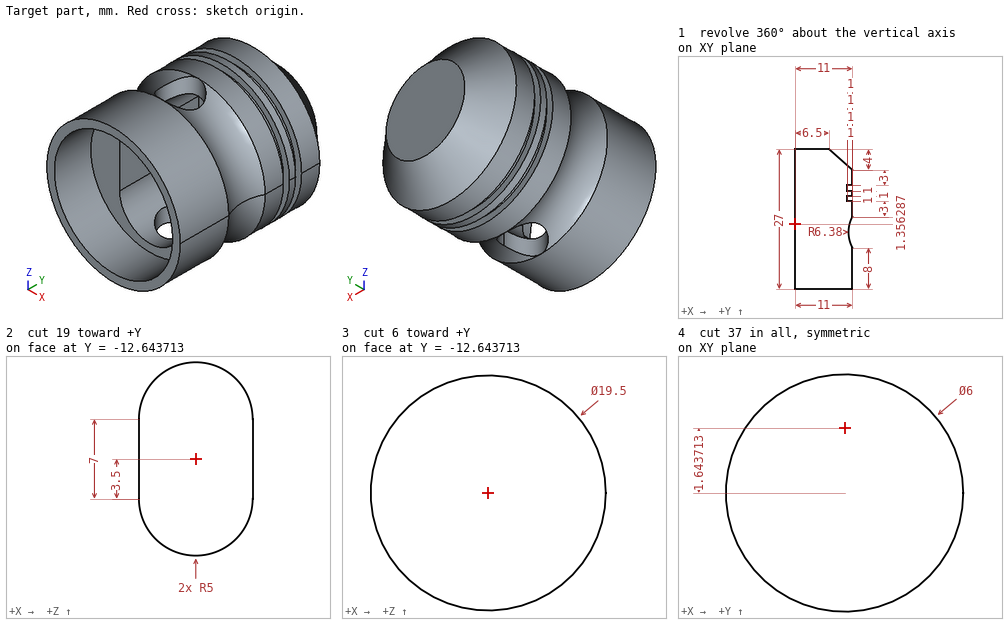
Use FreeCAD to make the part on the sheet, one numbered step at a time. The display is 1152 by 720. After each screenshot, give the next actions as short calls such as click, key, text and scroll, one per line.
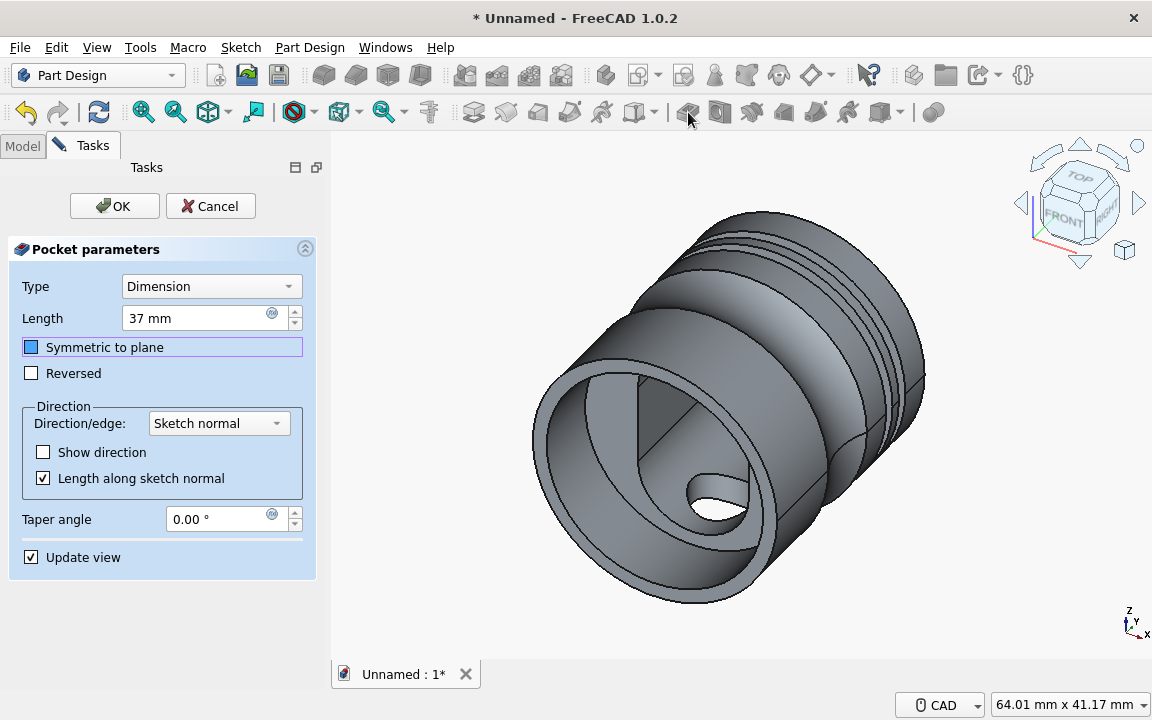
click(30, 347)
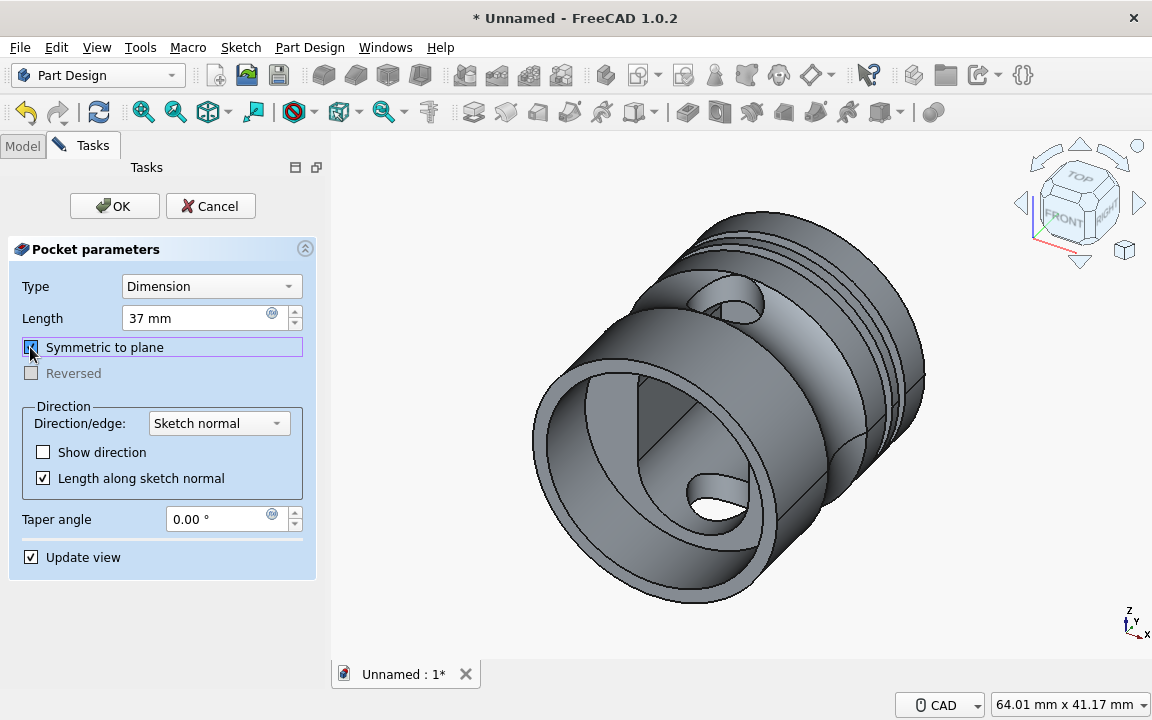
click(115, 206)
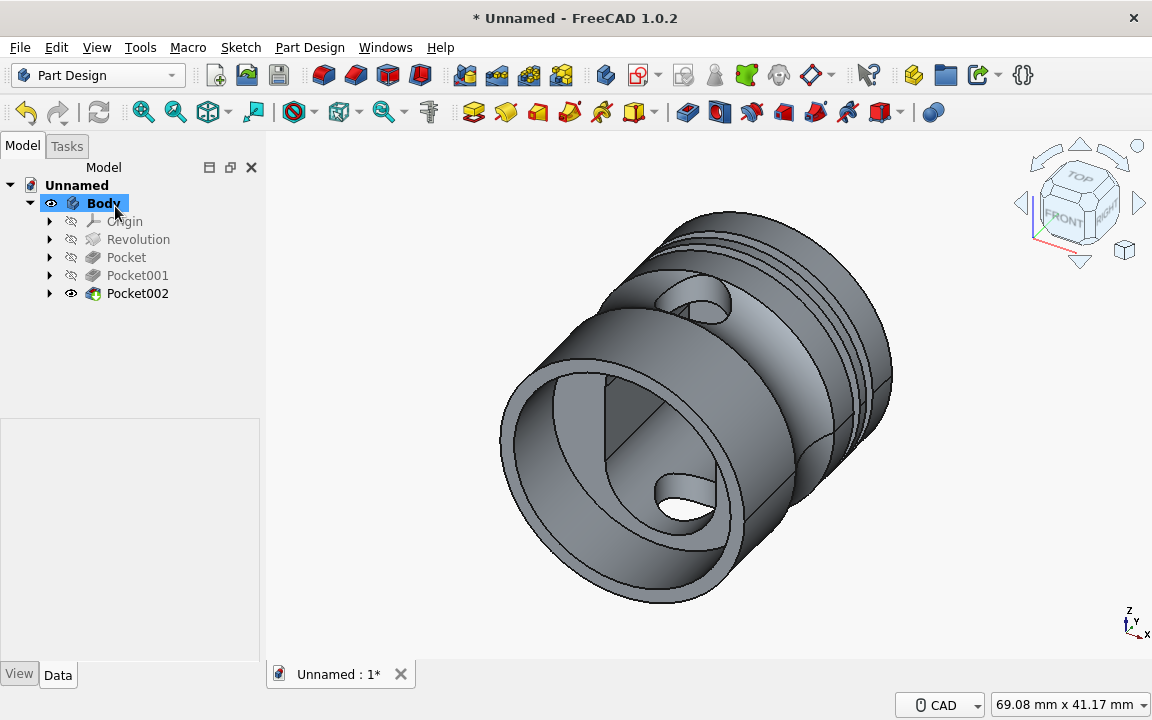
key(0)